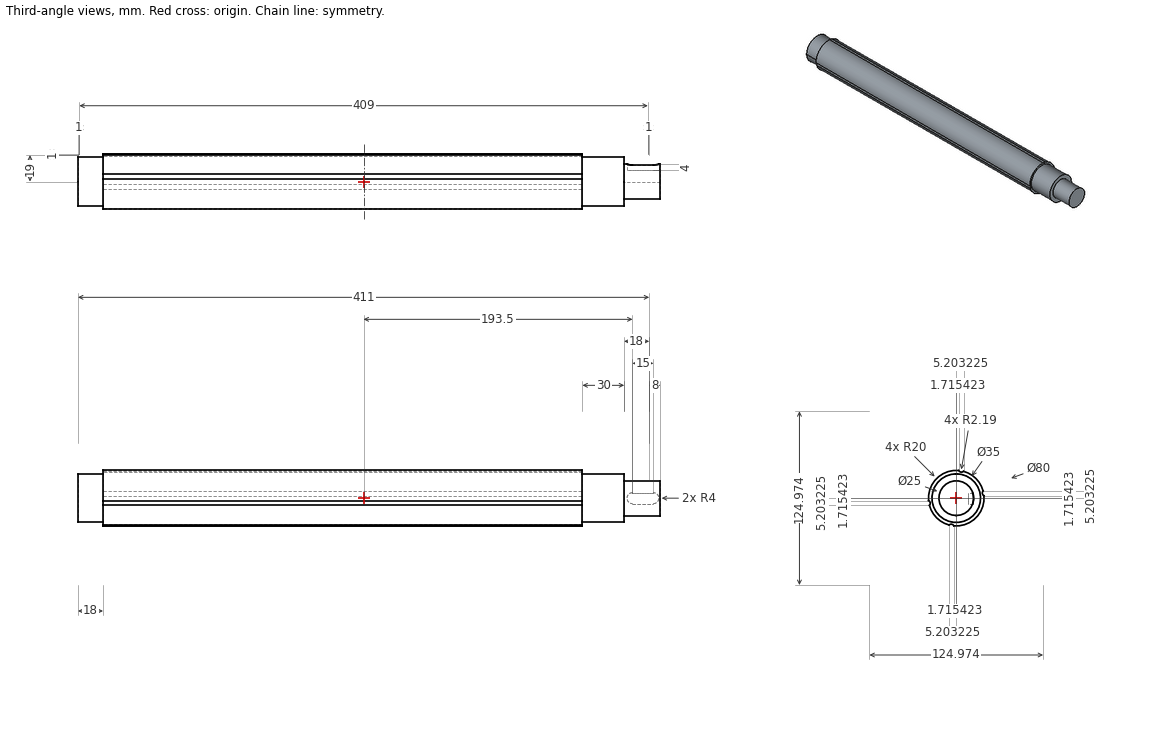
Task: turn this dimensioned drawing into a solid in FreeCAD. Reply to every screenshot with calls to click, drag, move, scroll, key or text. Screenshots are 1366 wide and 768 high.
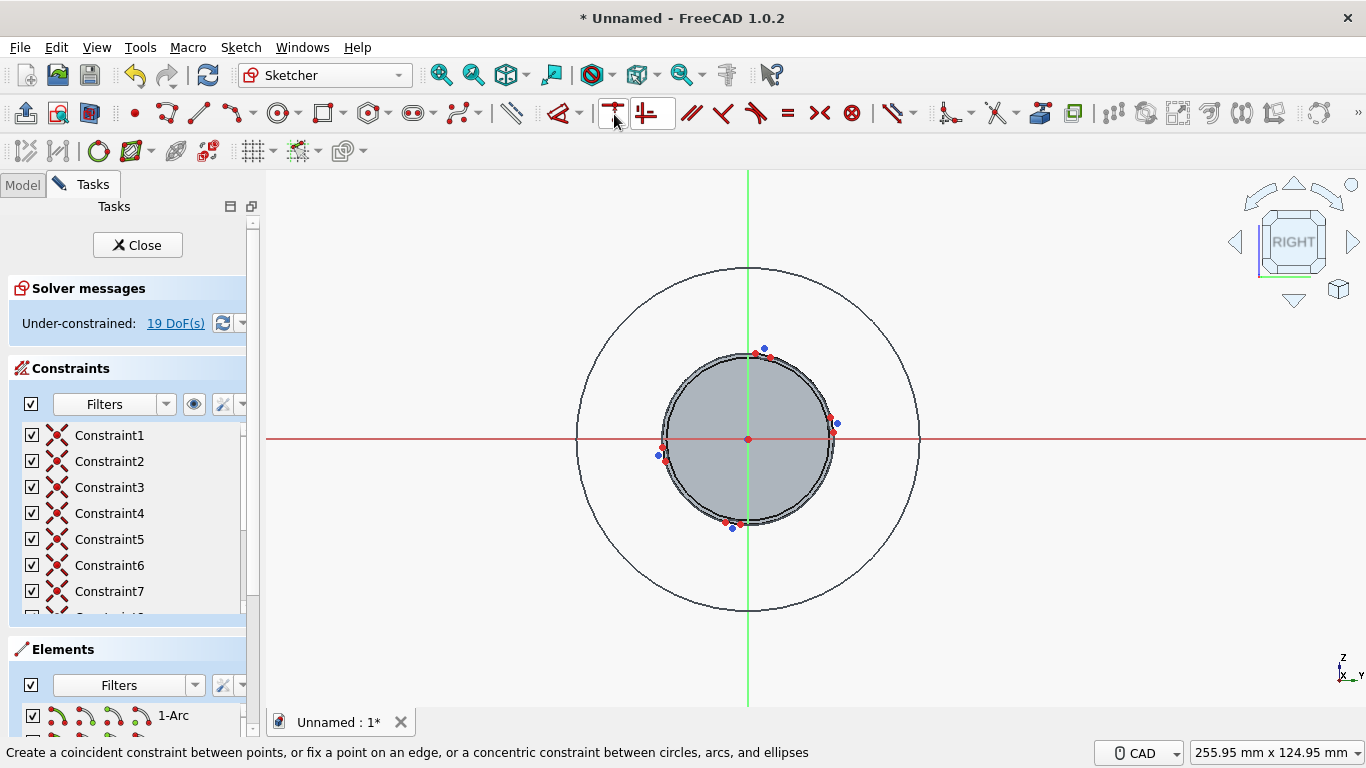
scroll(748, 439, up, 8)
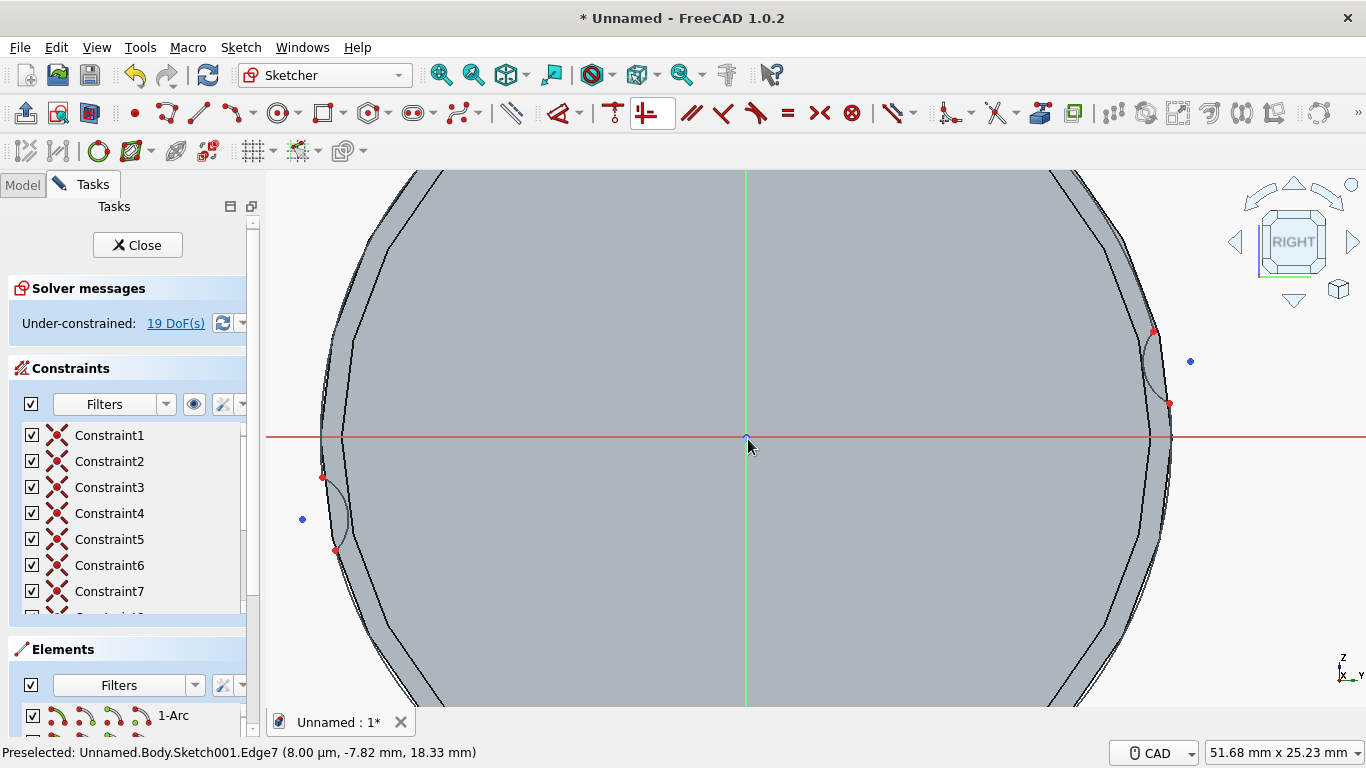
drag(736, 427, 757, 450)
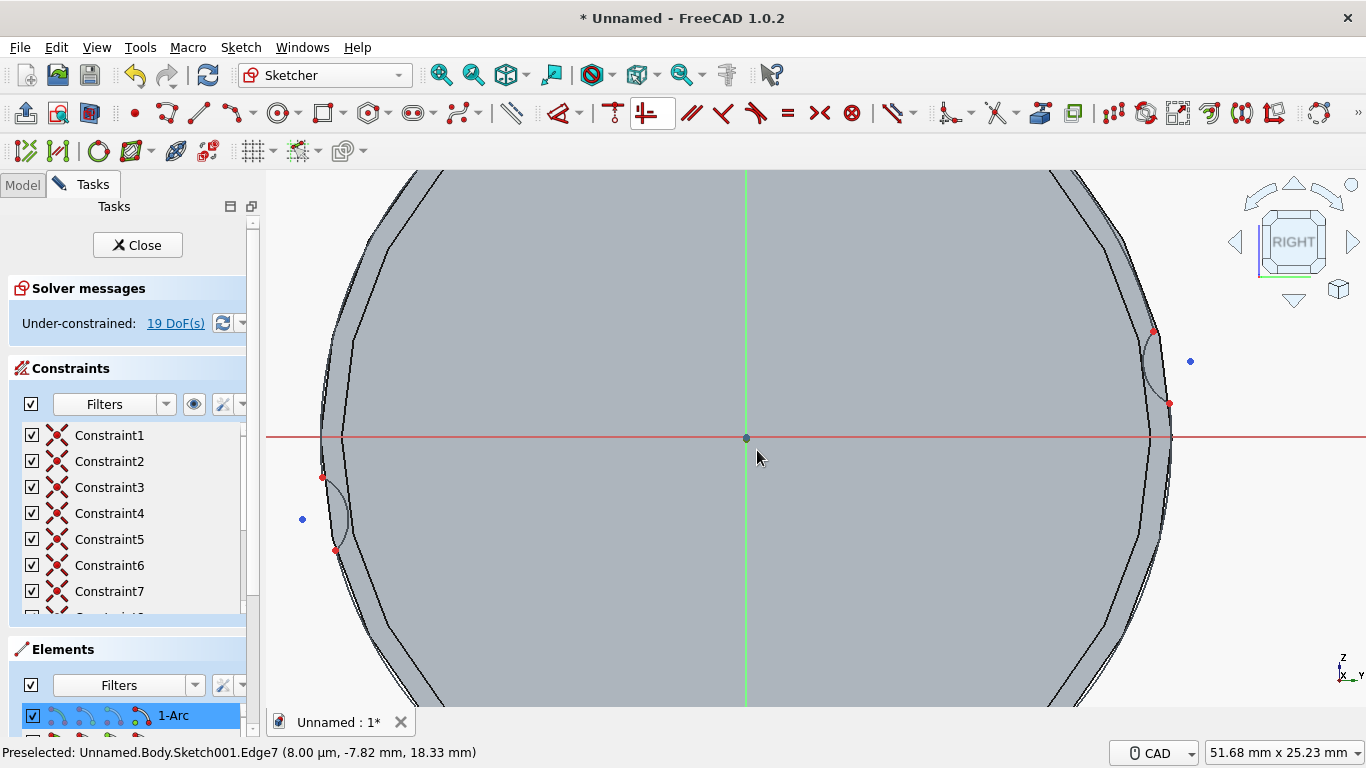
key(c)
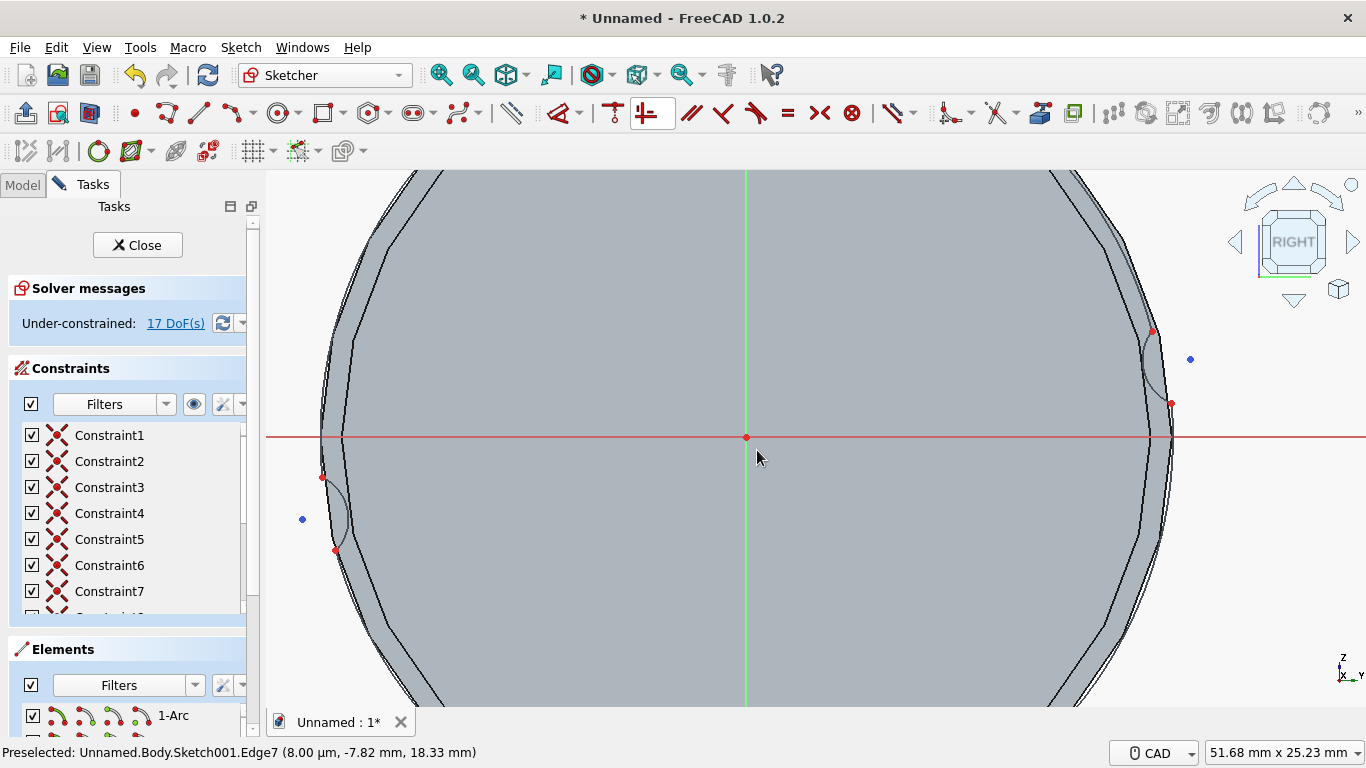
scroll(748, 439, down, 8)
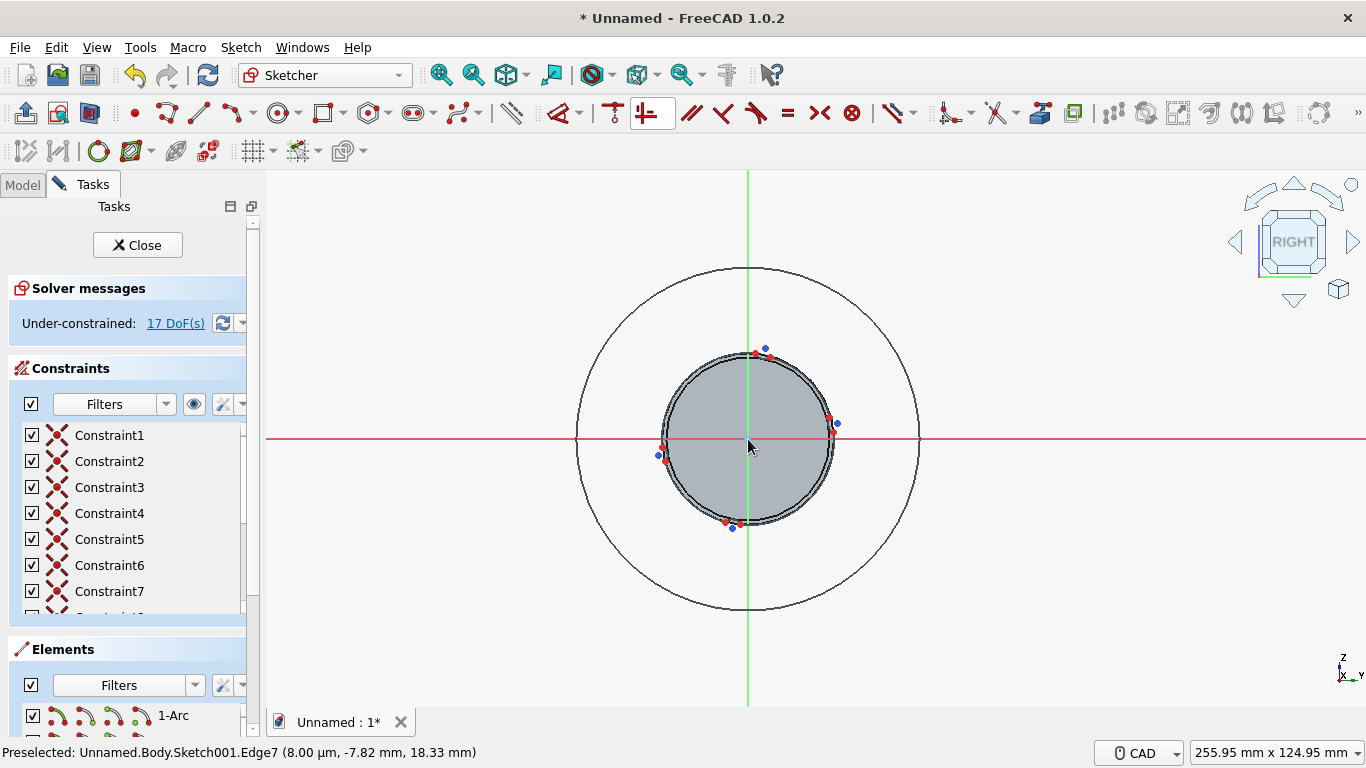
click(819, 393)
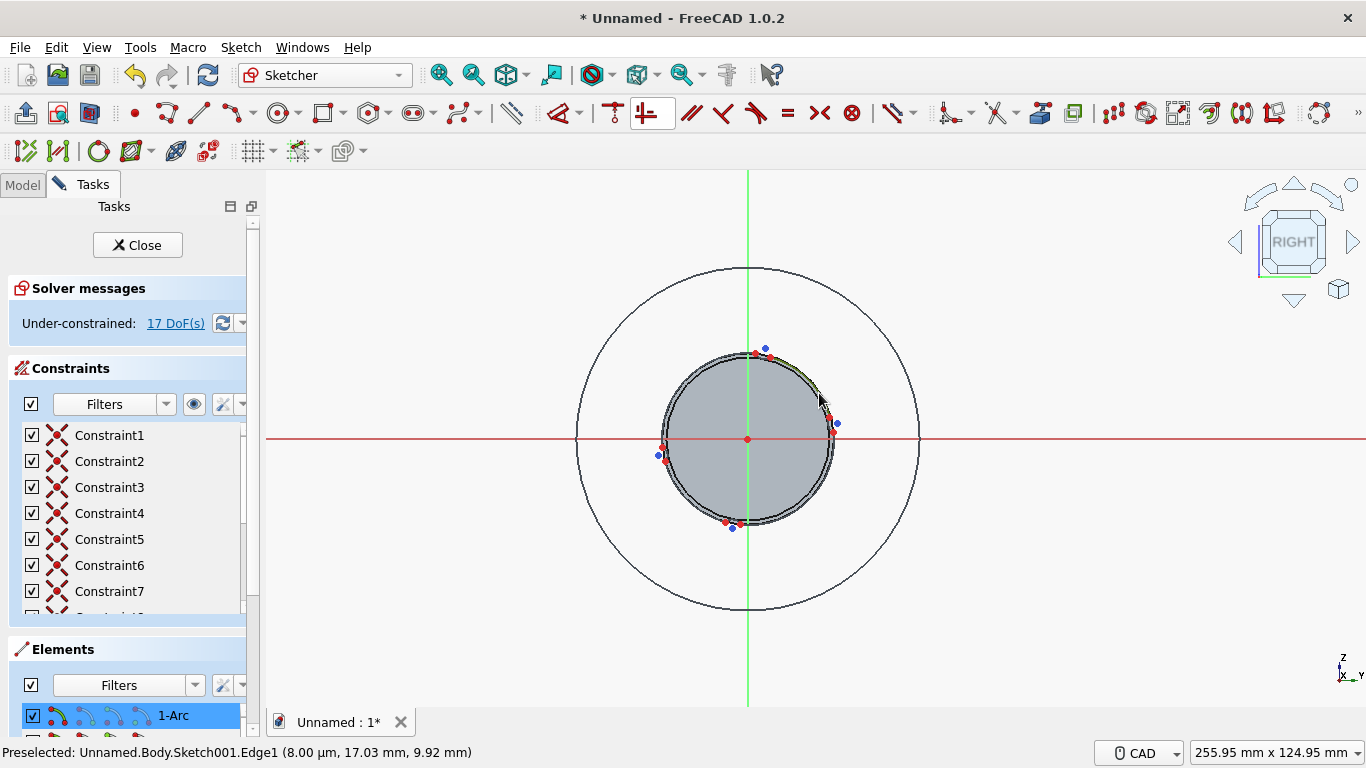
click(784, 517)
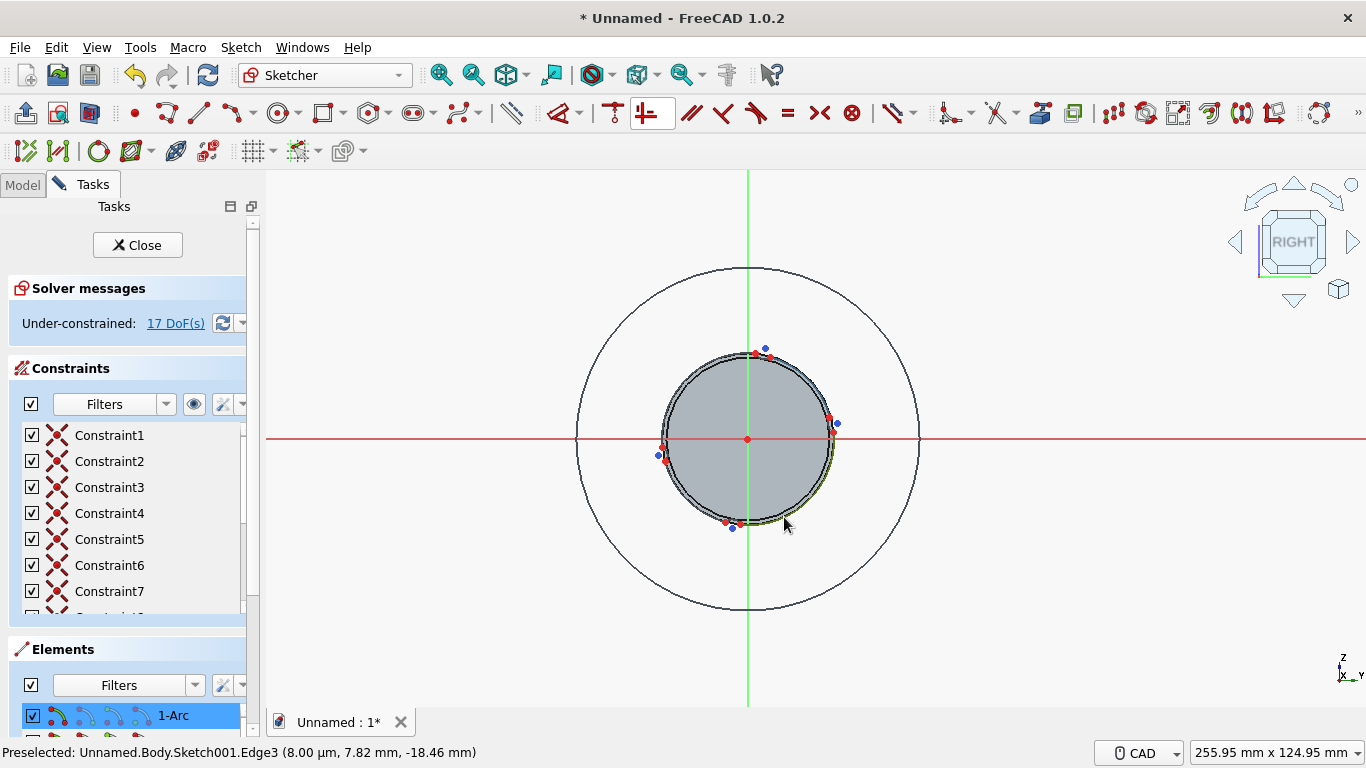
click(676, 486)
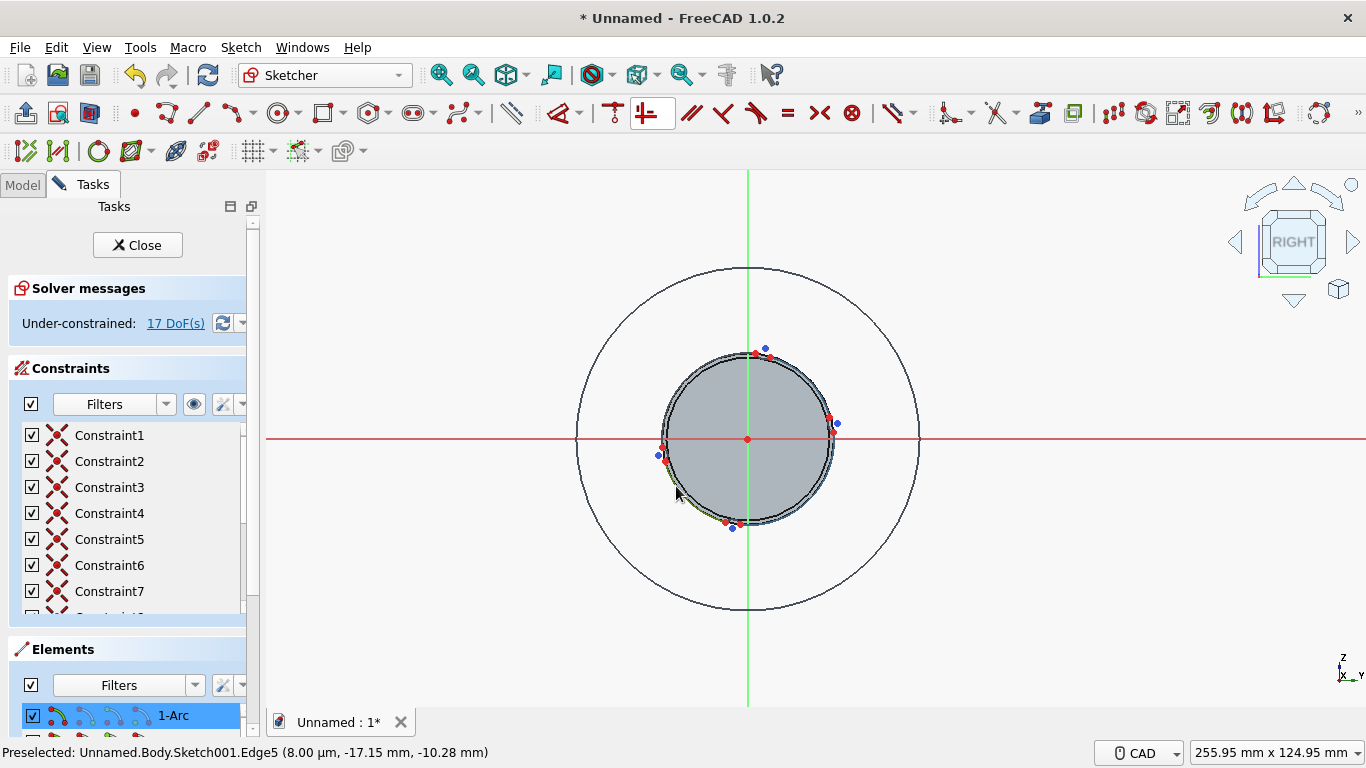
click(712, 361)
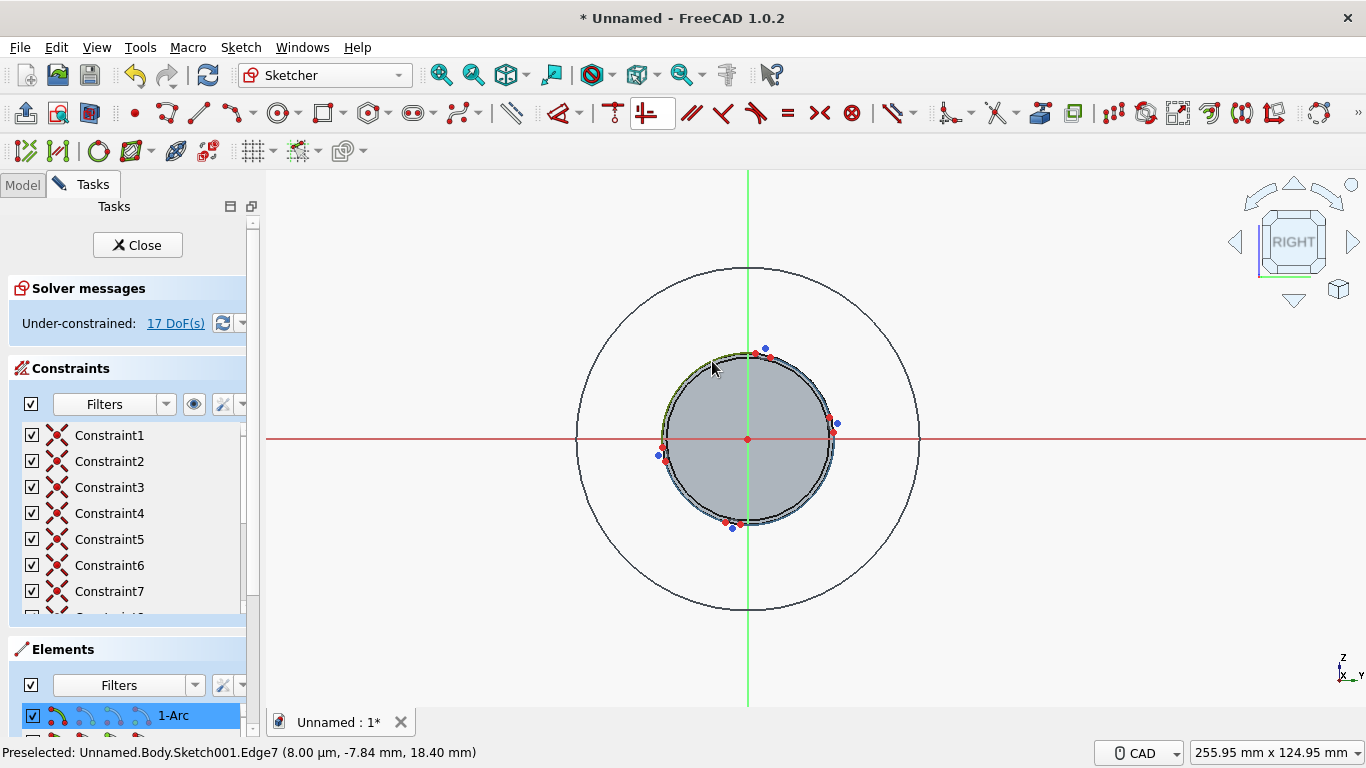
click(788, 114)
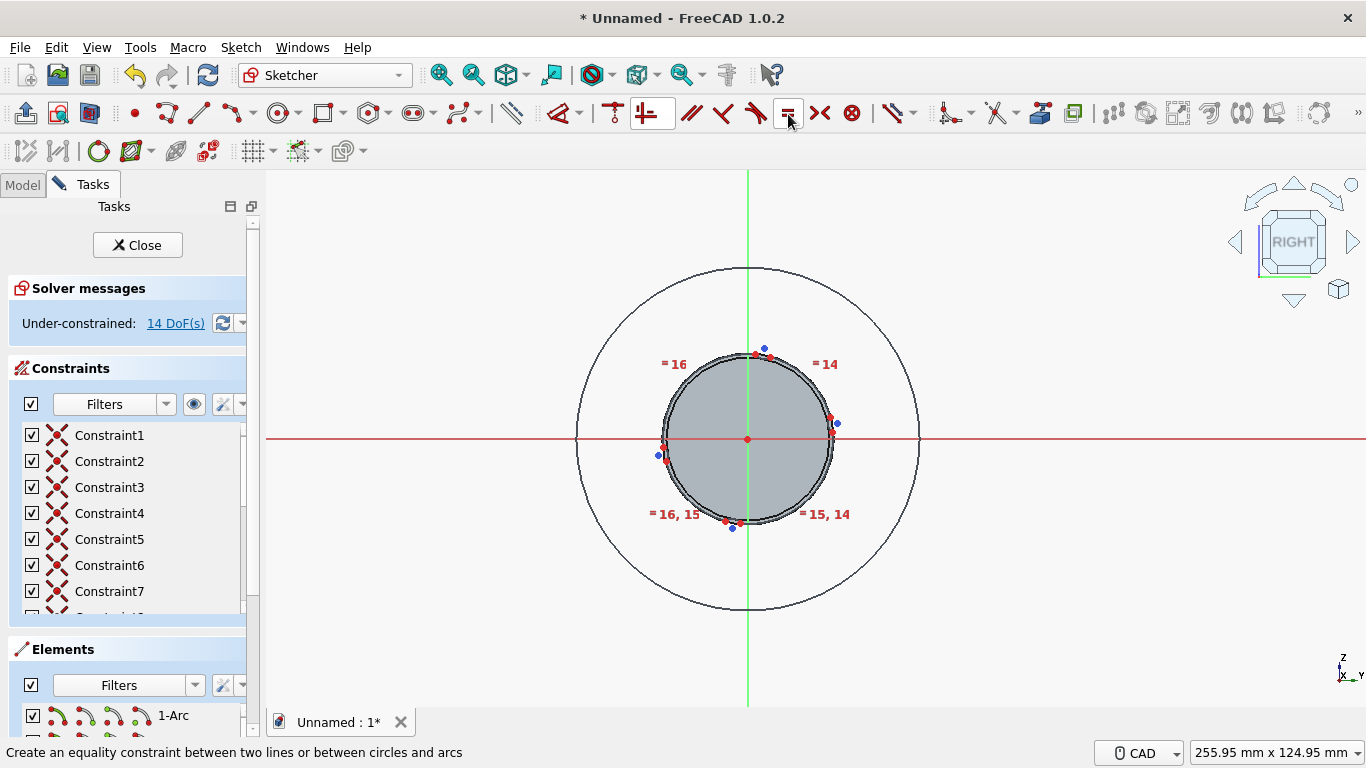
scroll(828, 425, up, 3)